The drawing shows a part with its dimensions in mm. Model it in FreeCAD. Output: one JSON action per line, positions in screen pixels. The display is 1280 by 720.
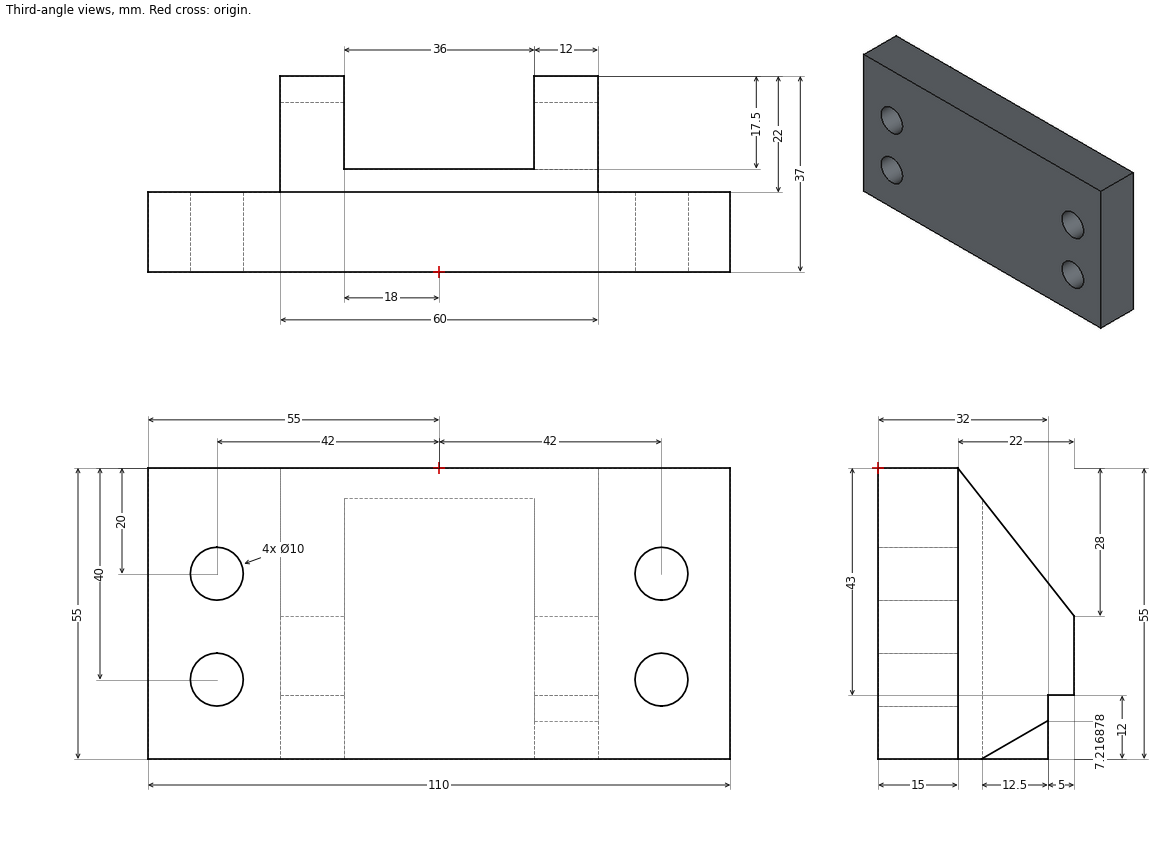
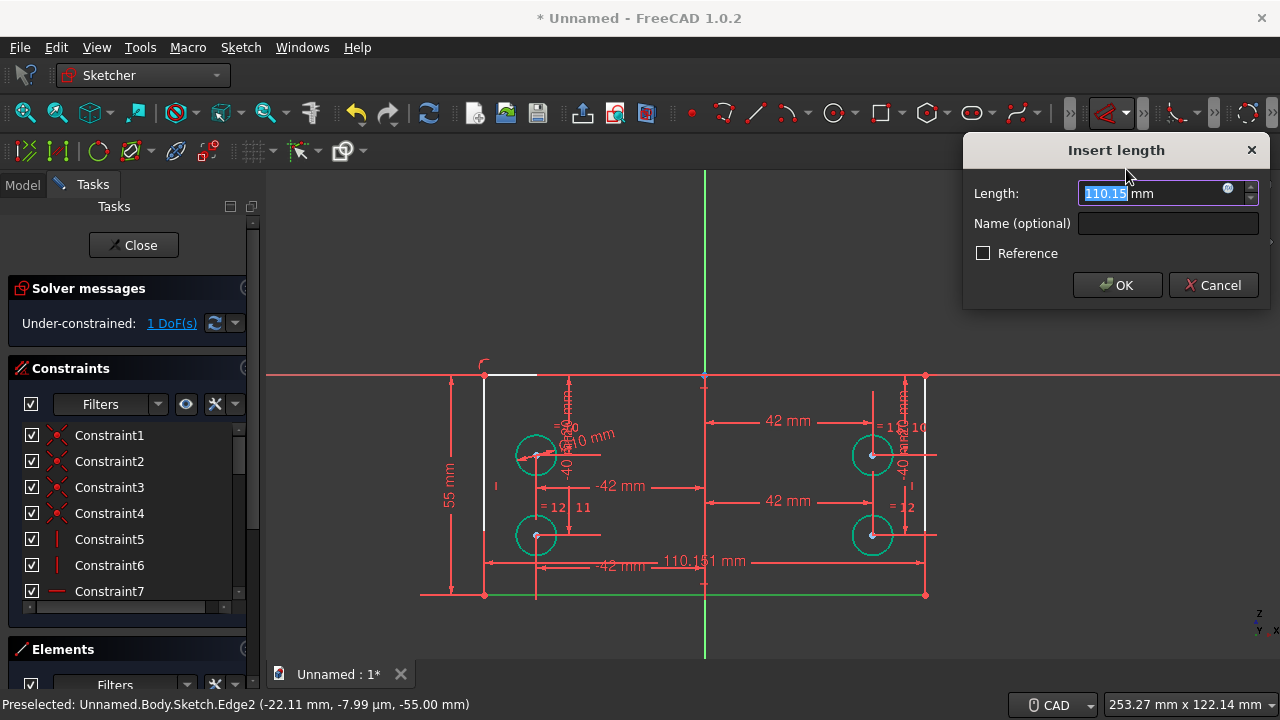
{"action": "type", "text": "110"}
{"action": "key", "text": "Return"}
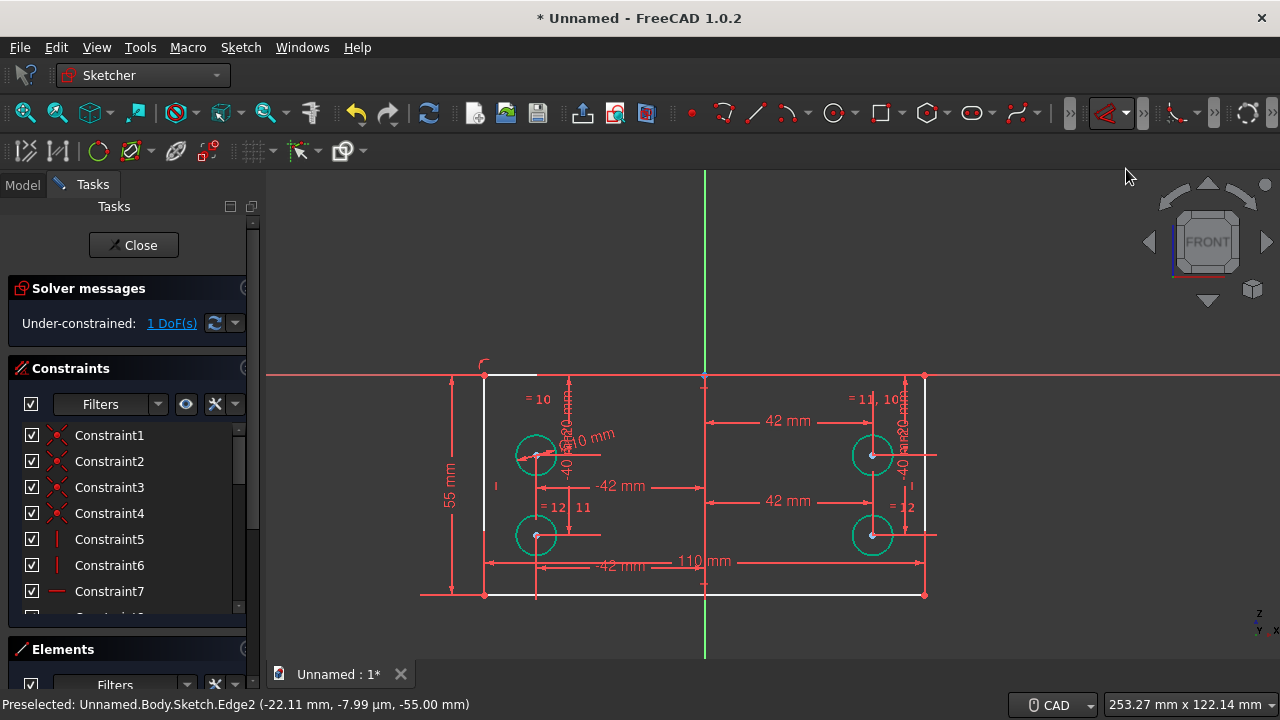
{"action": "left_click", "coordinate": [484, 375]}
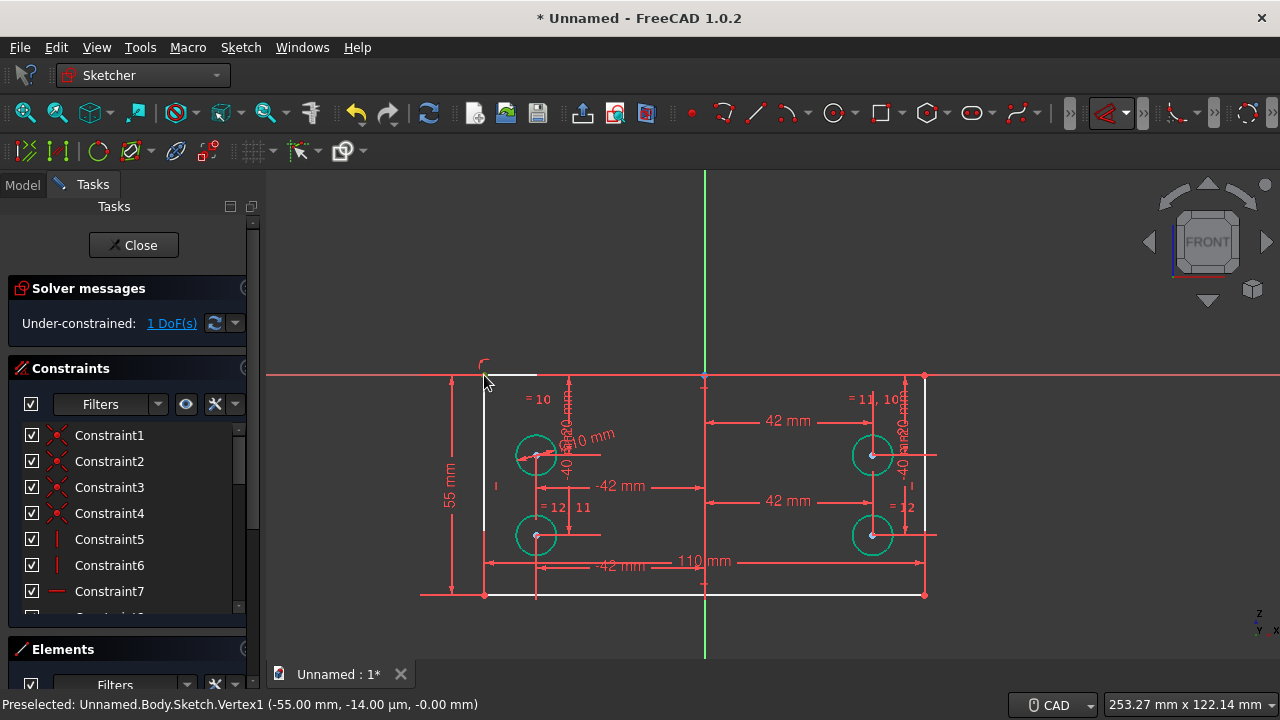
{"action": "left_click", "coordinate": [1128, 114]}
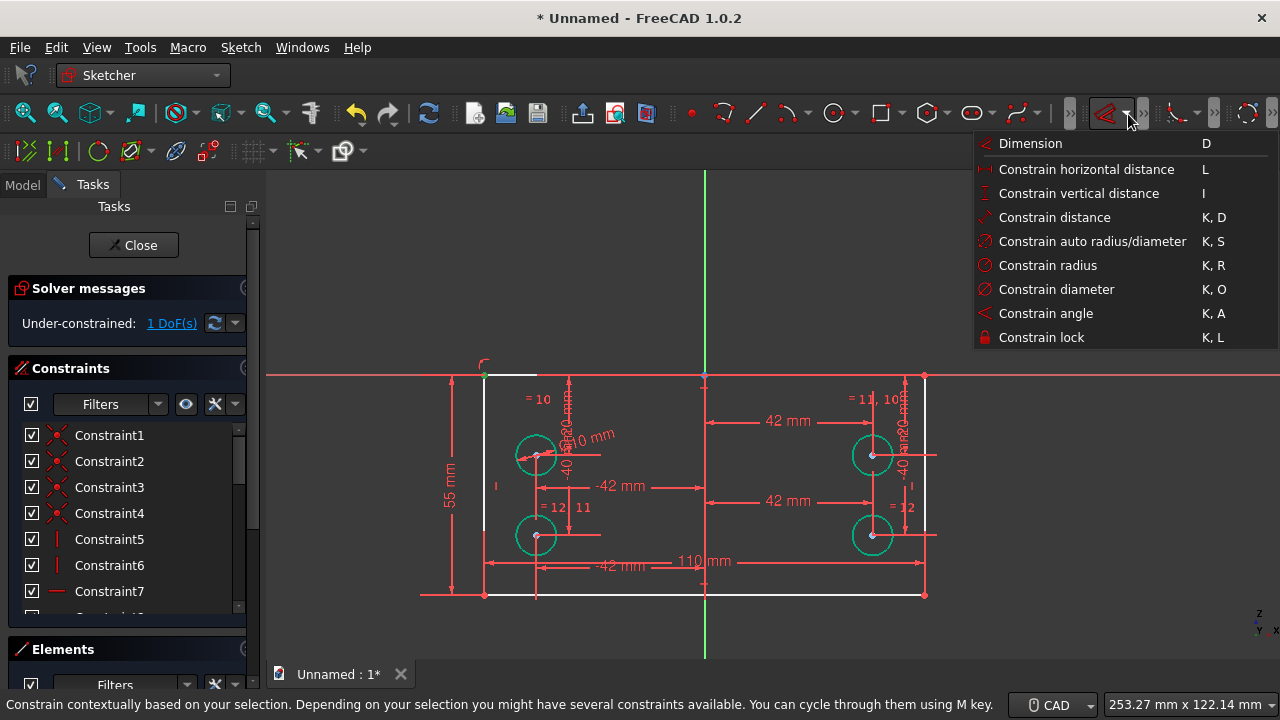
{"action": "left_click", "coordinate": [1126, 169]}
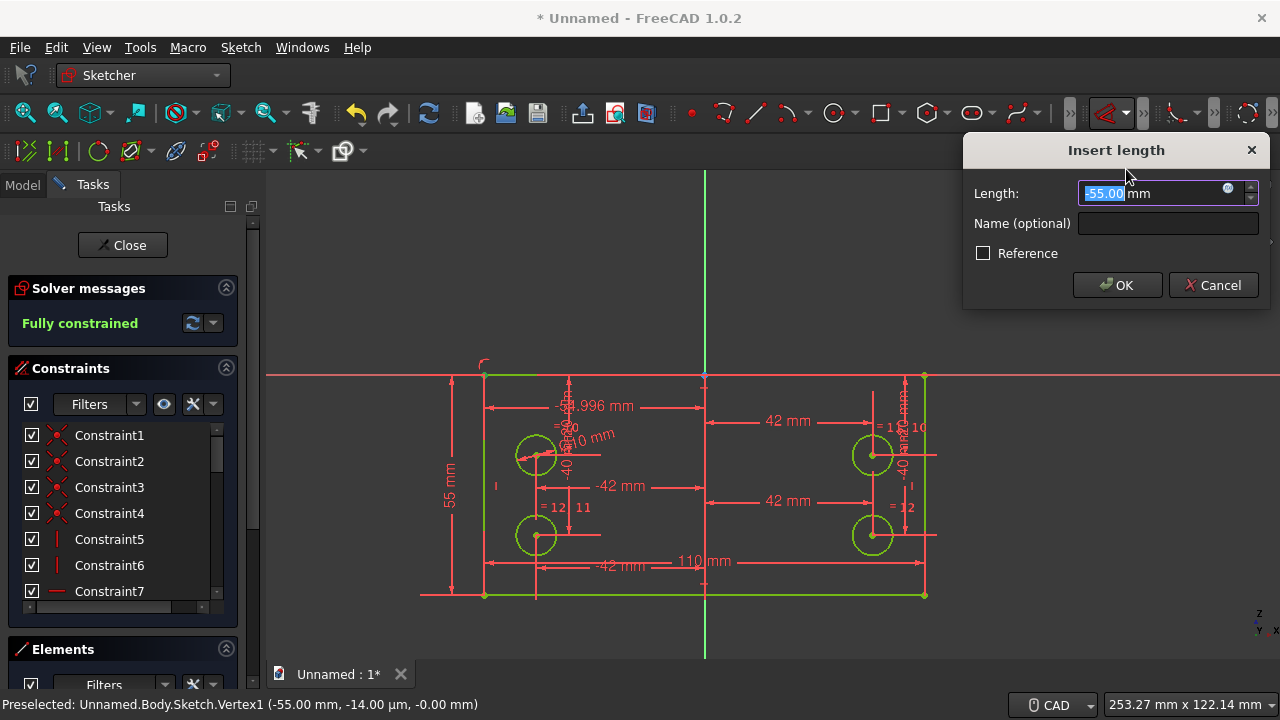
{"action": "type", "text": "-55"}
{"action": "key", "text": "Return"}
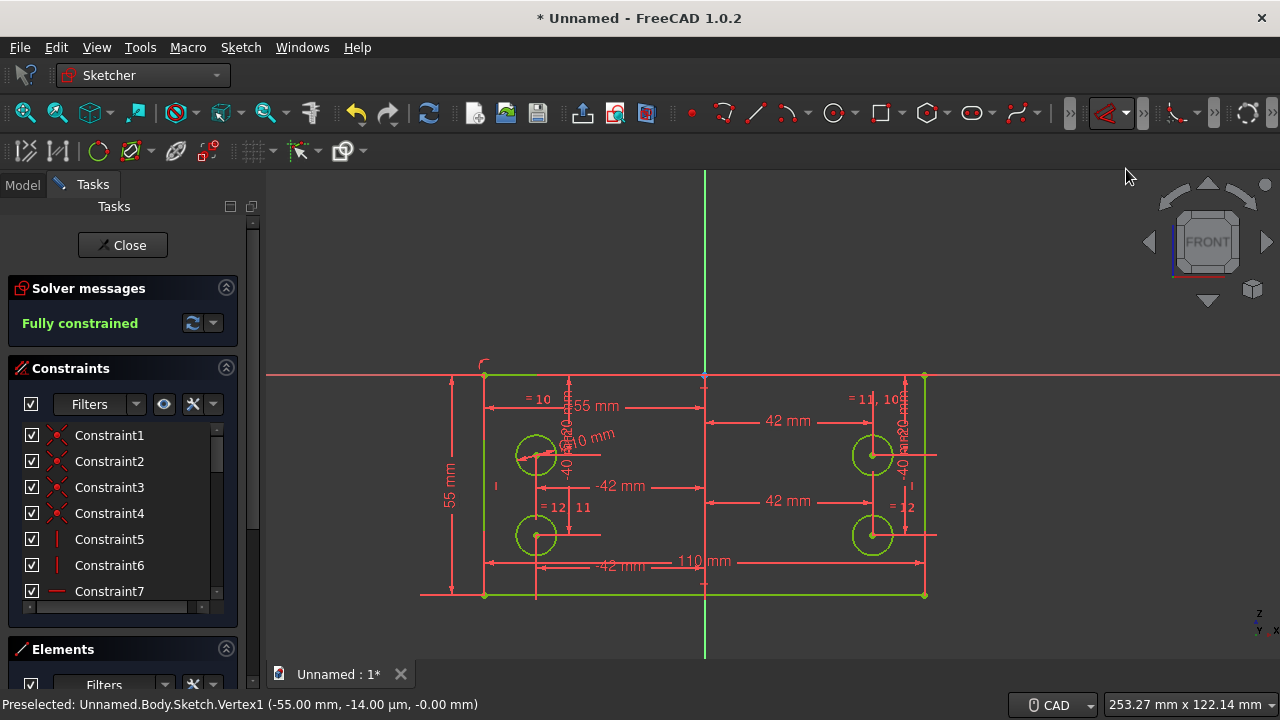
{"action": "left_click", "coordinate": [123, 245]}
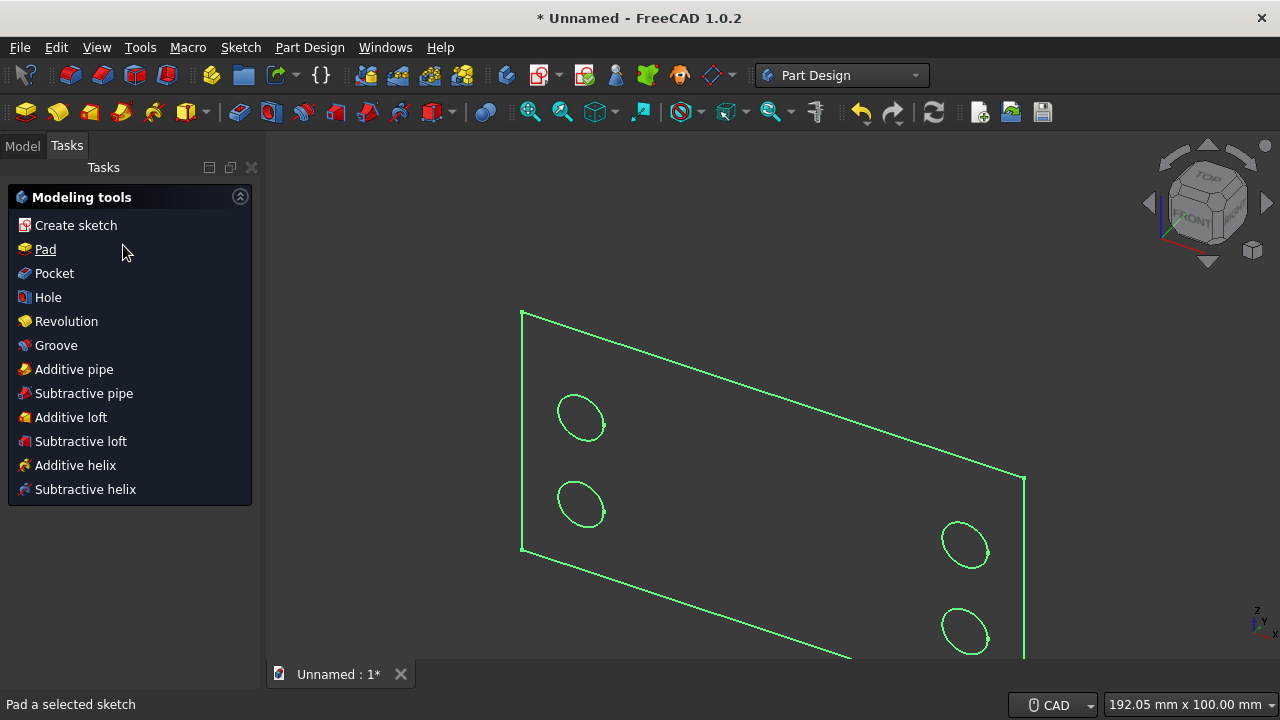
{"action": "left_click", "coordinate": [26, 112]}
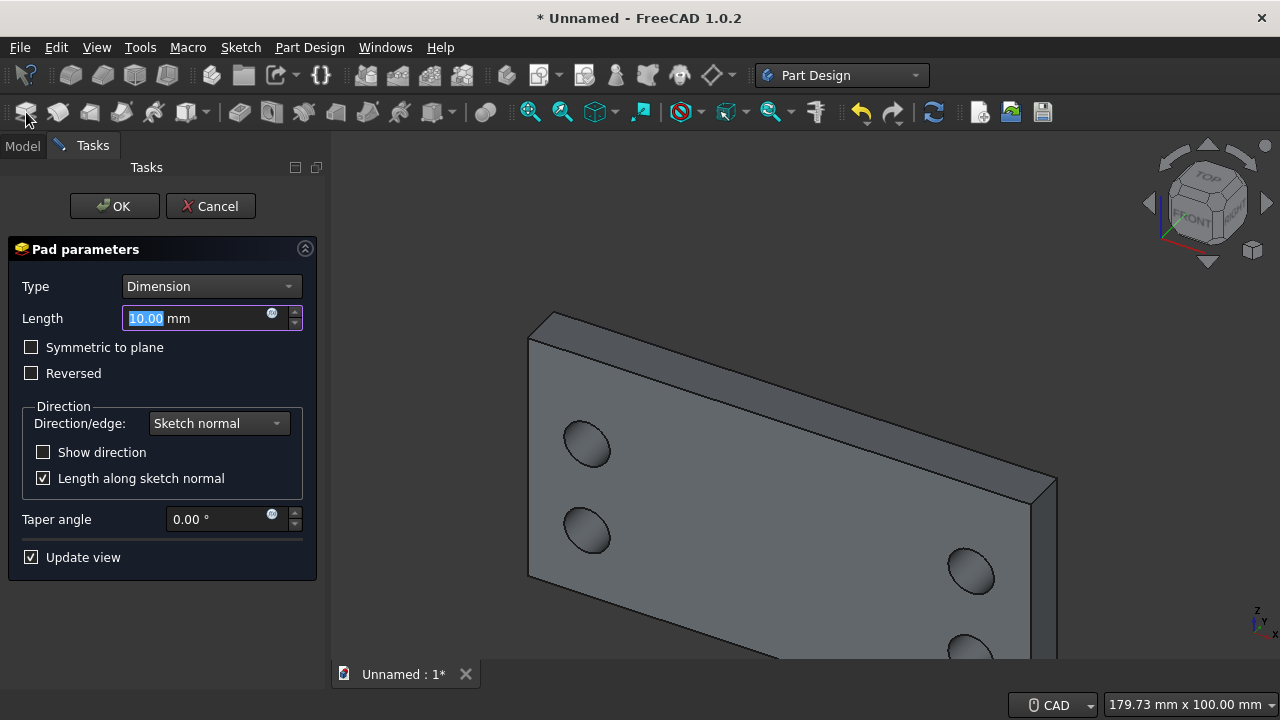
{"action": "type", "text": "15"}
{"action": "key", "text": "Tab"}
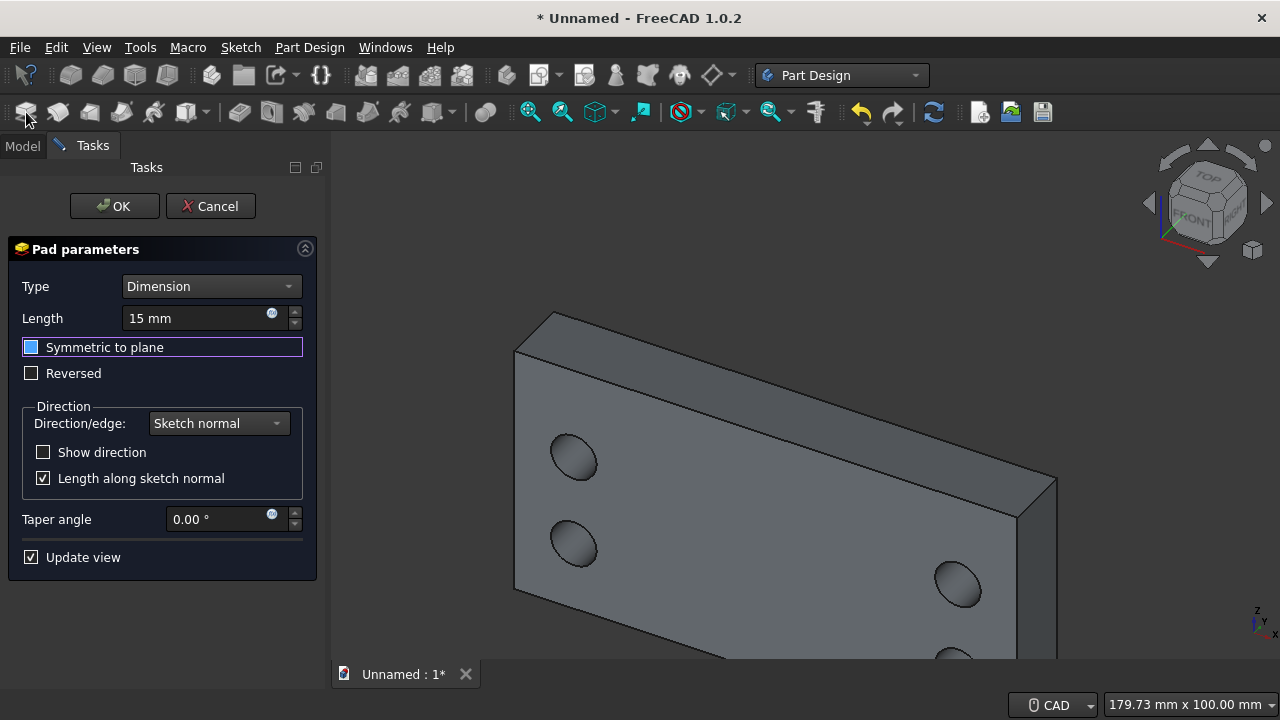
{"action": "left_click", "coordinate": [30, 373]}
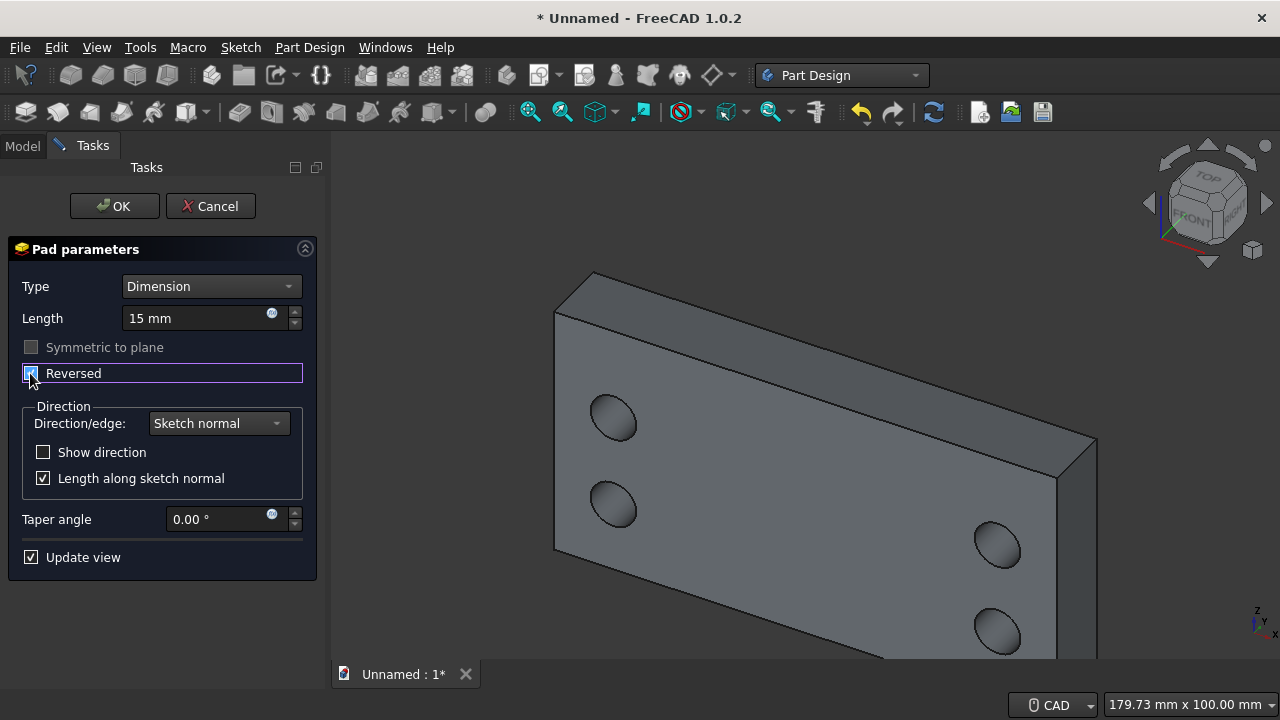
{"action": "left_click", "coordinate": [115, 206]}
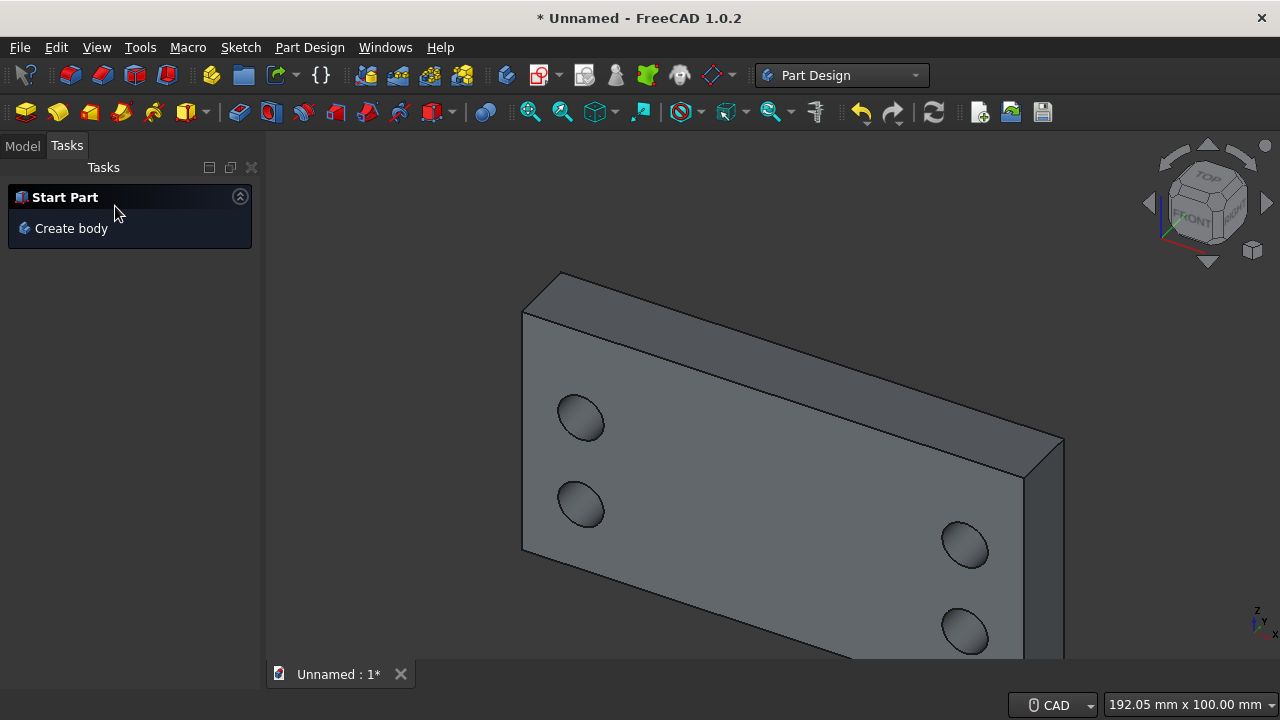
{"action": "left_click", "coordinate": [532, 112]}